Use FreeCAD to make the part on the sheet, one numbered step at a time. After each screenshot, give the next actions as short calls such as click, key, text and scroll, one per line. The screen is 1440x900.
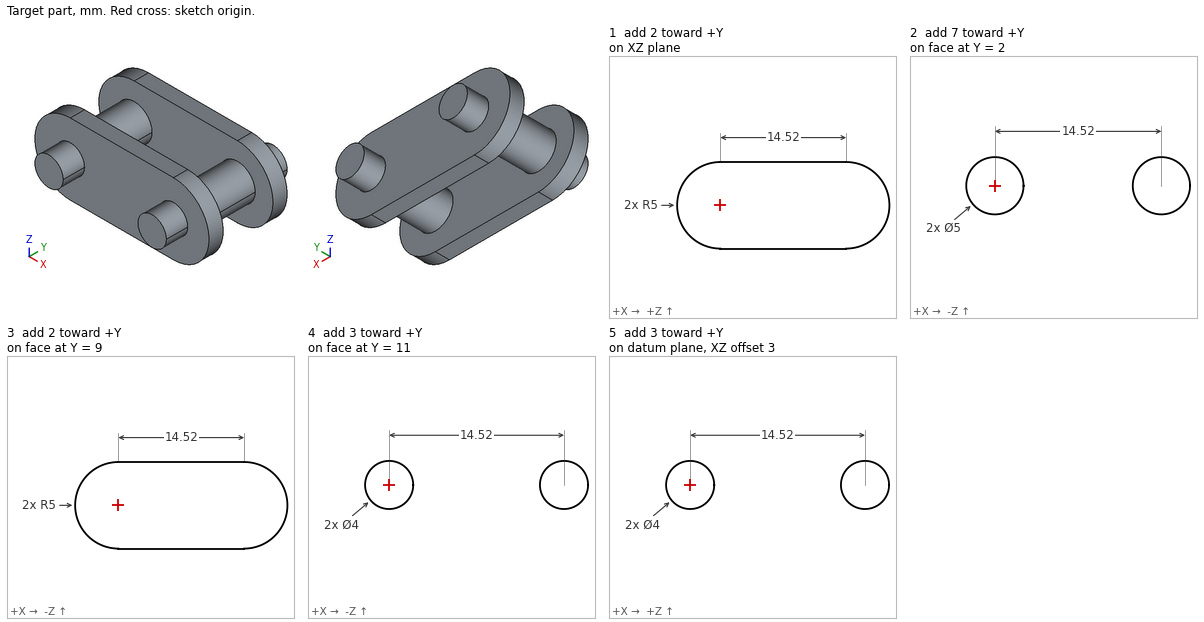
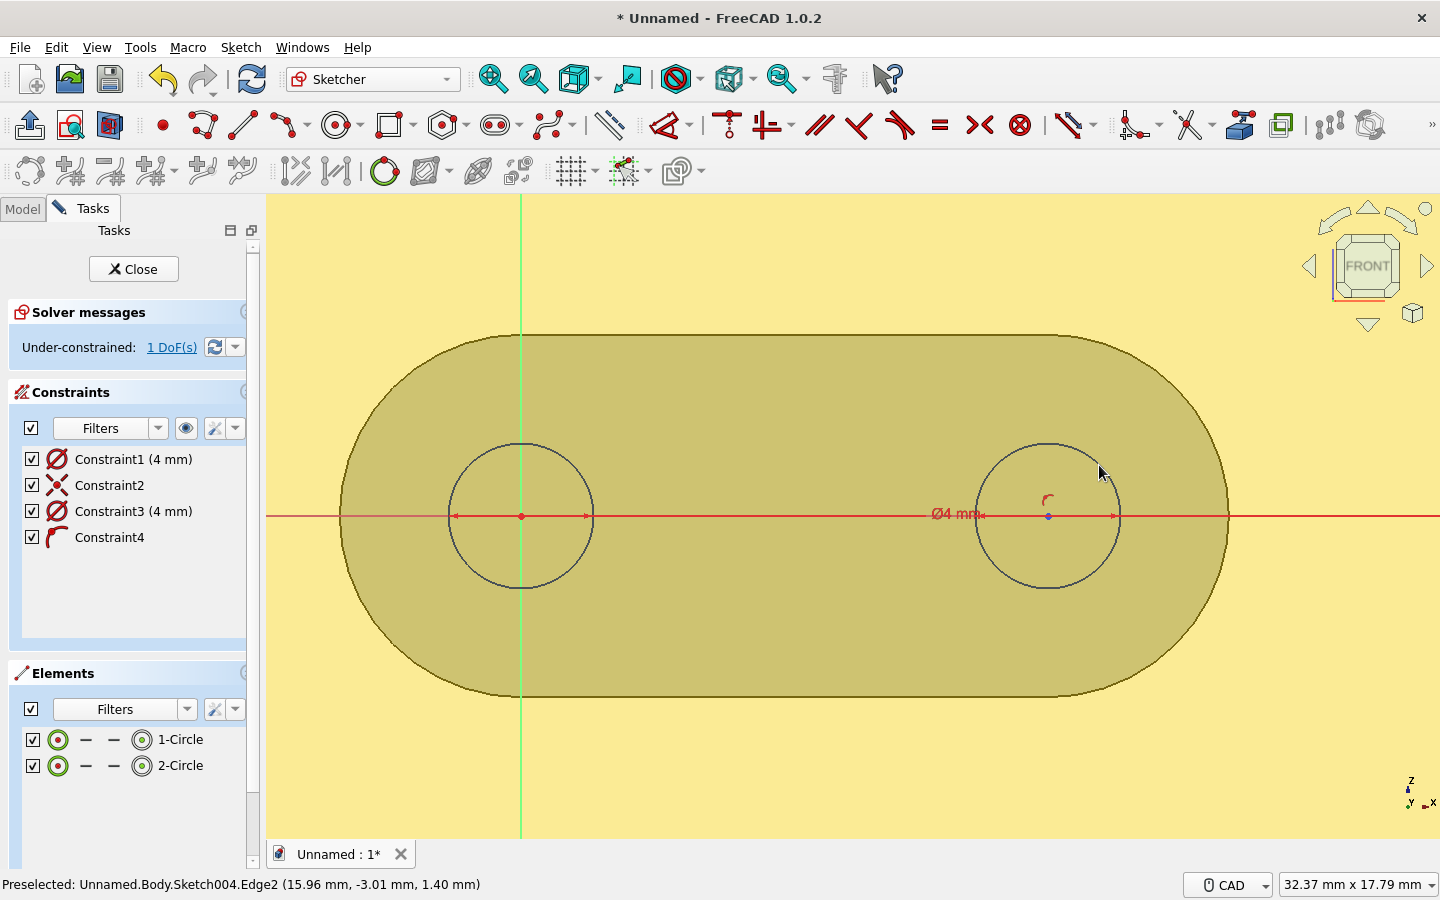
key(d)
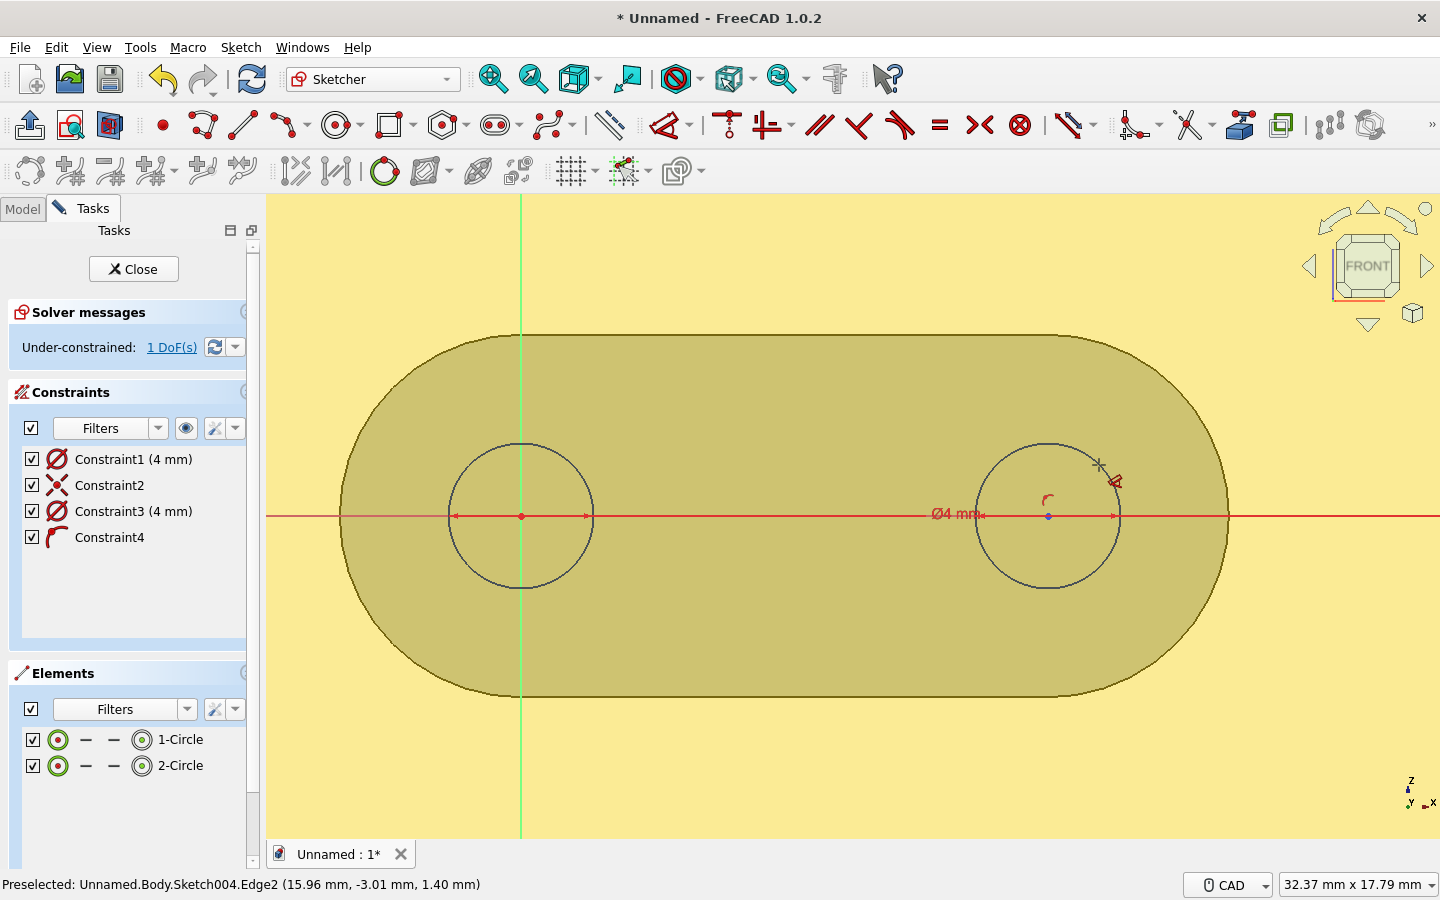
click(1048, 516)
click(785, 550)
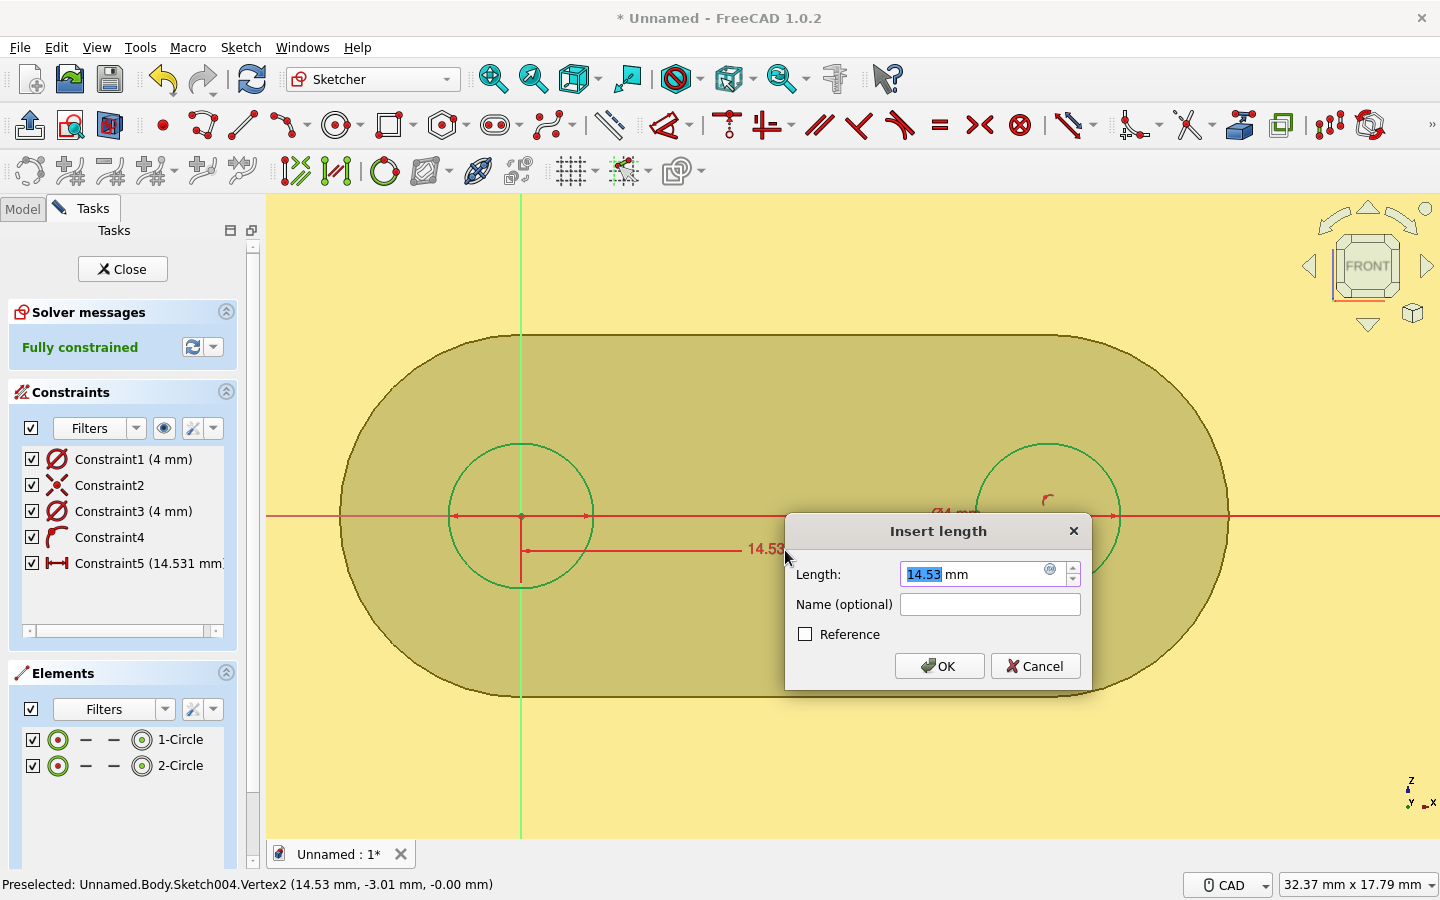
text(14.52)
key(Return)
key(Escape)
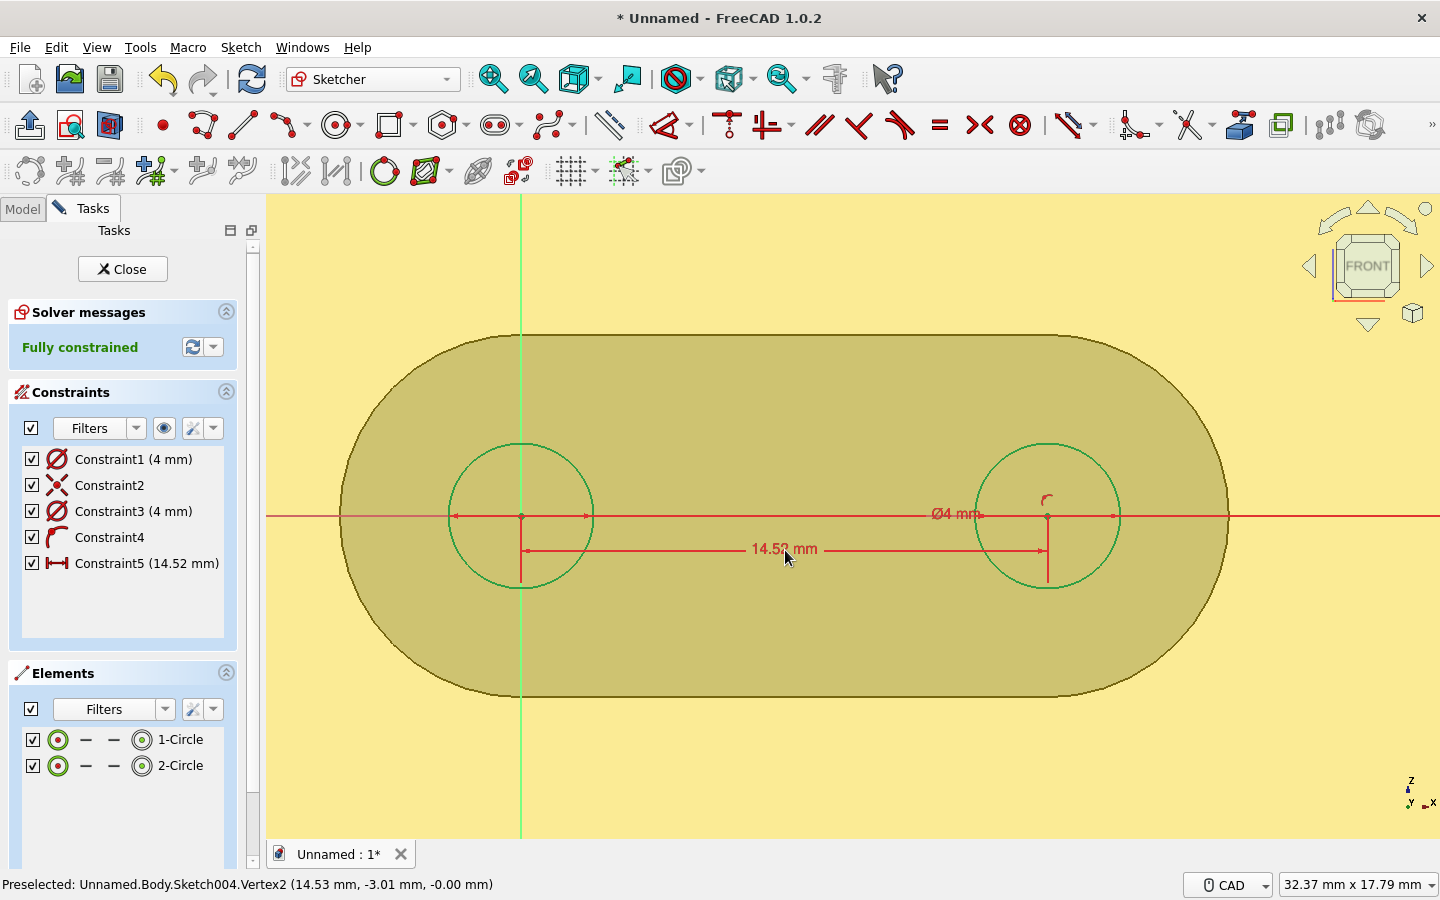
click(123, 269)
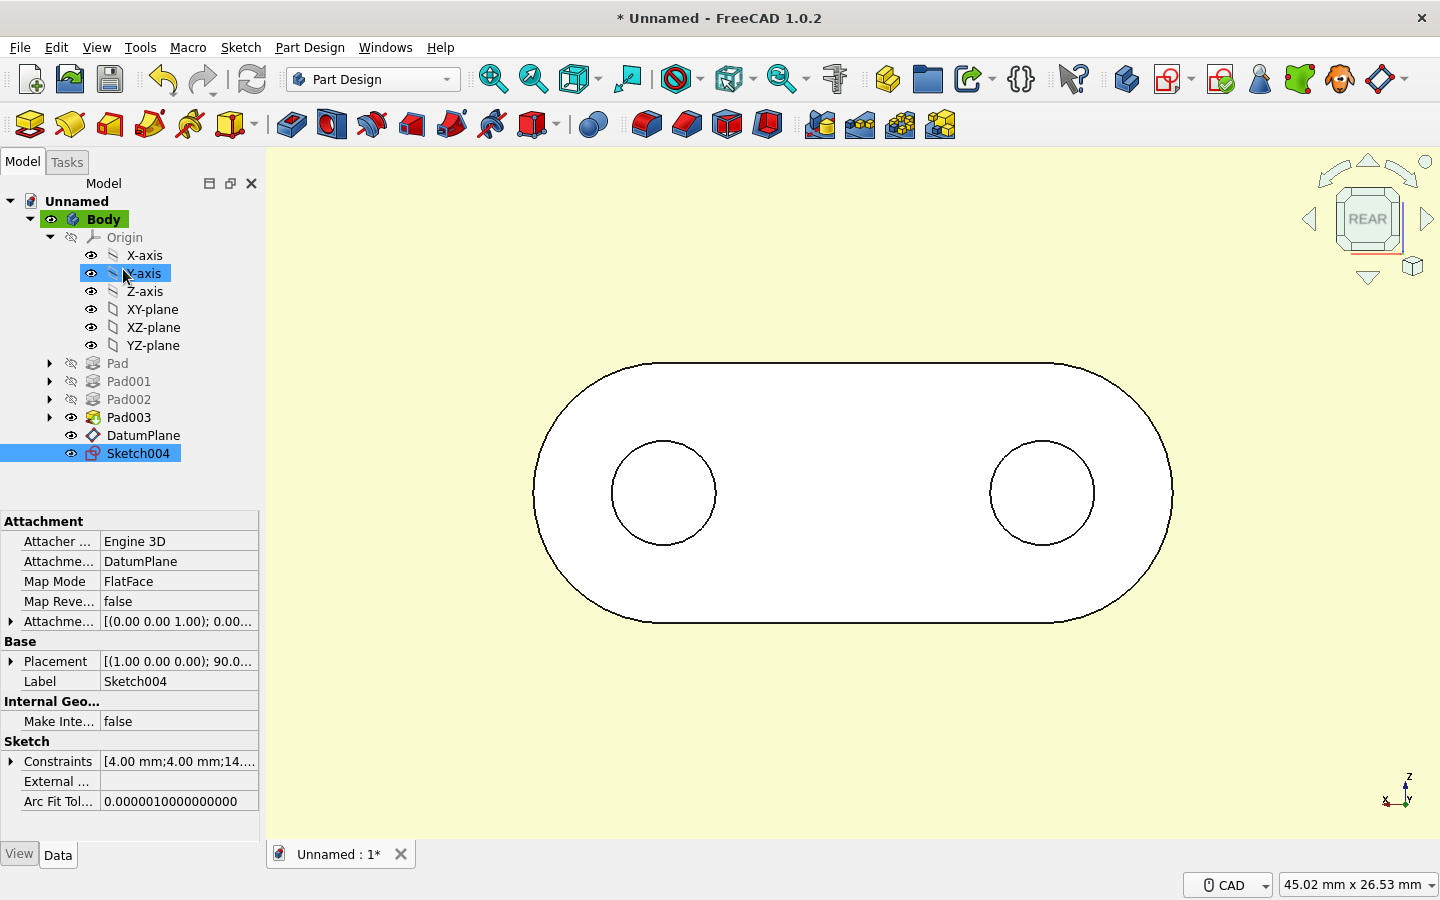
click(30, 124)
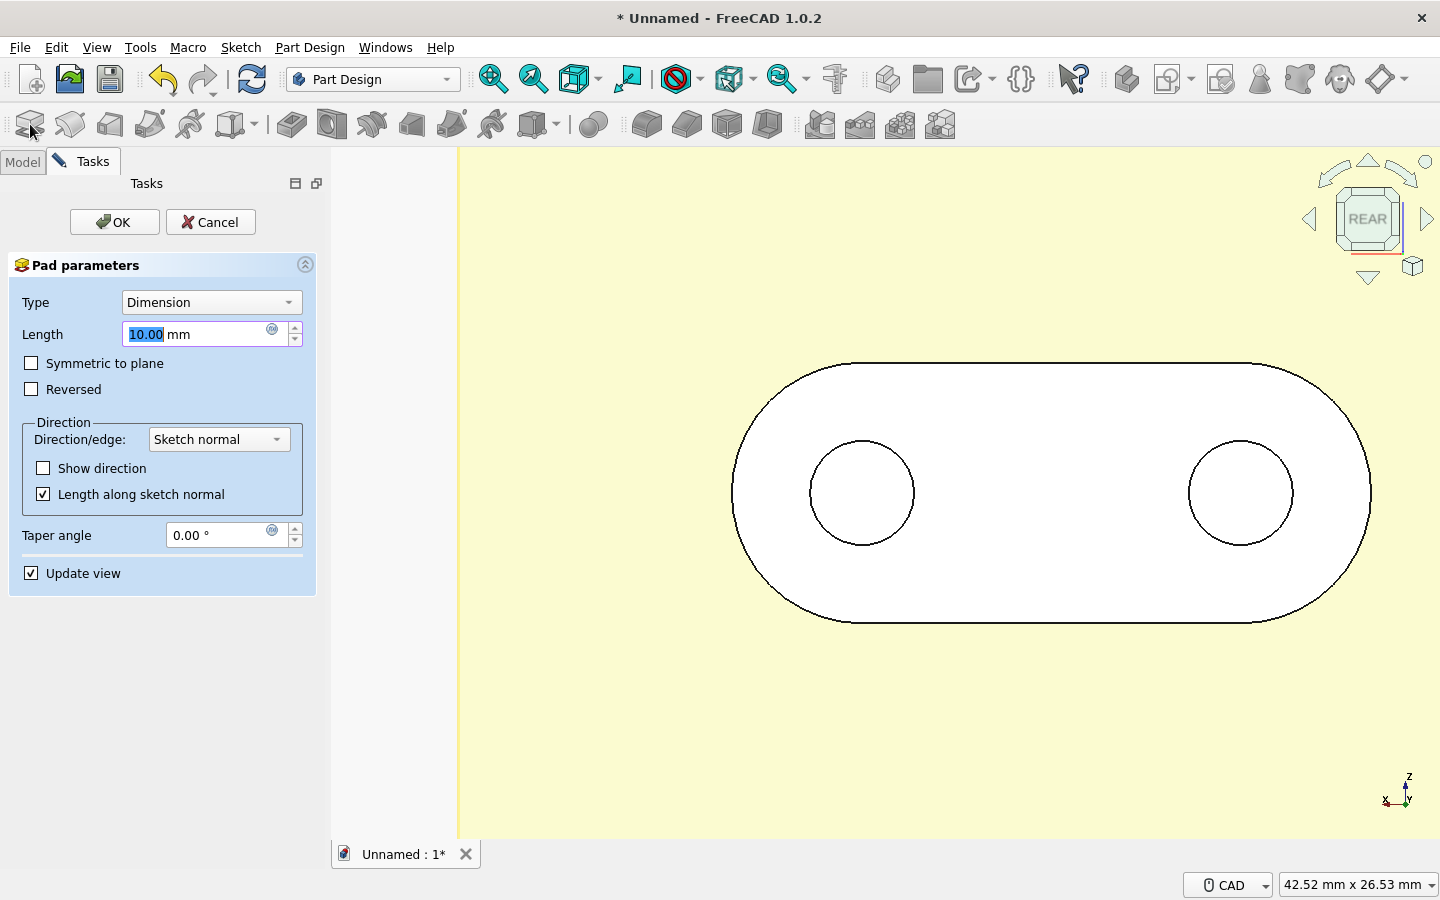
text(3)
key(Tab)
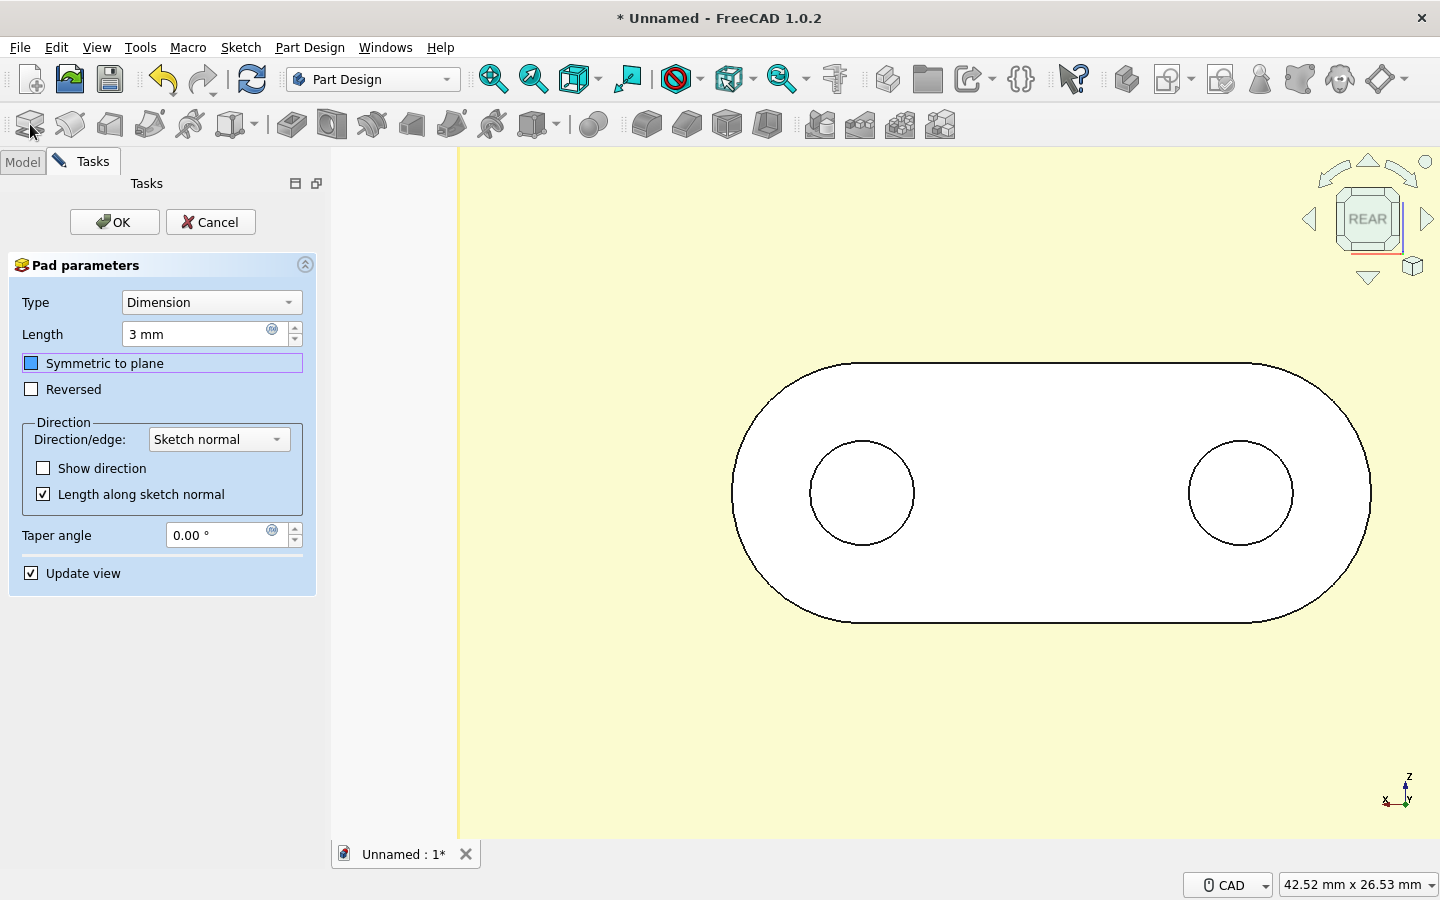
click(30, 389)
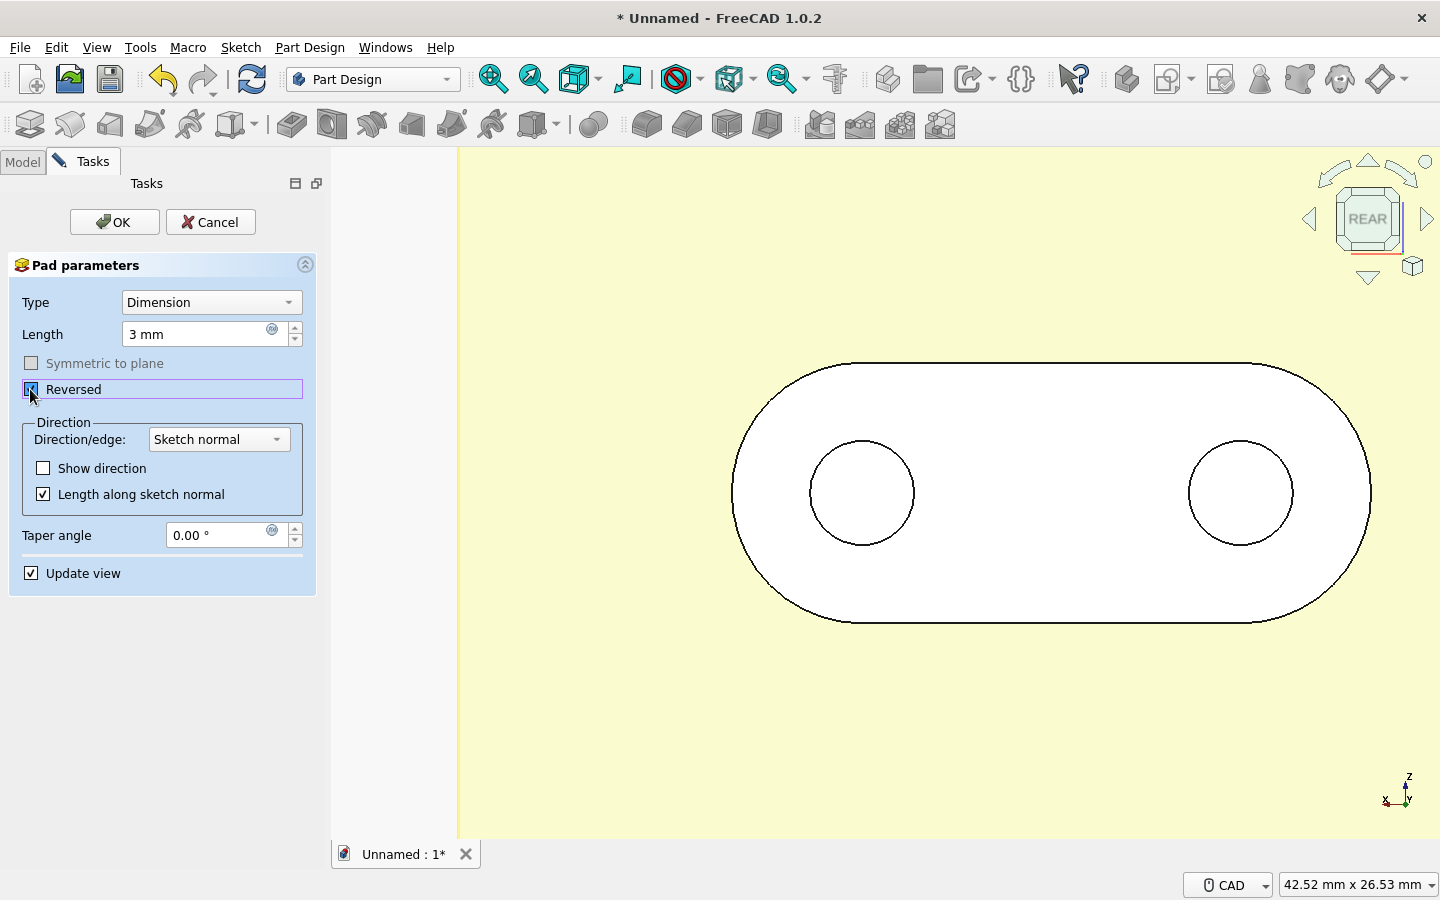
click(115, 222)